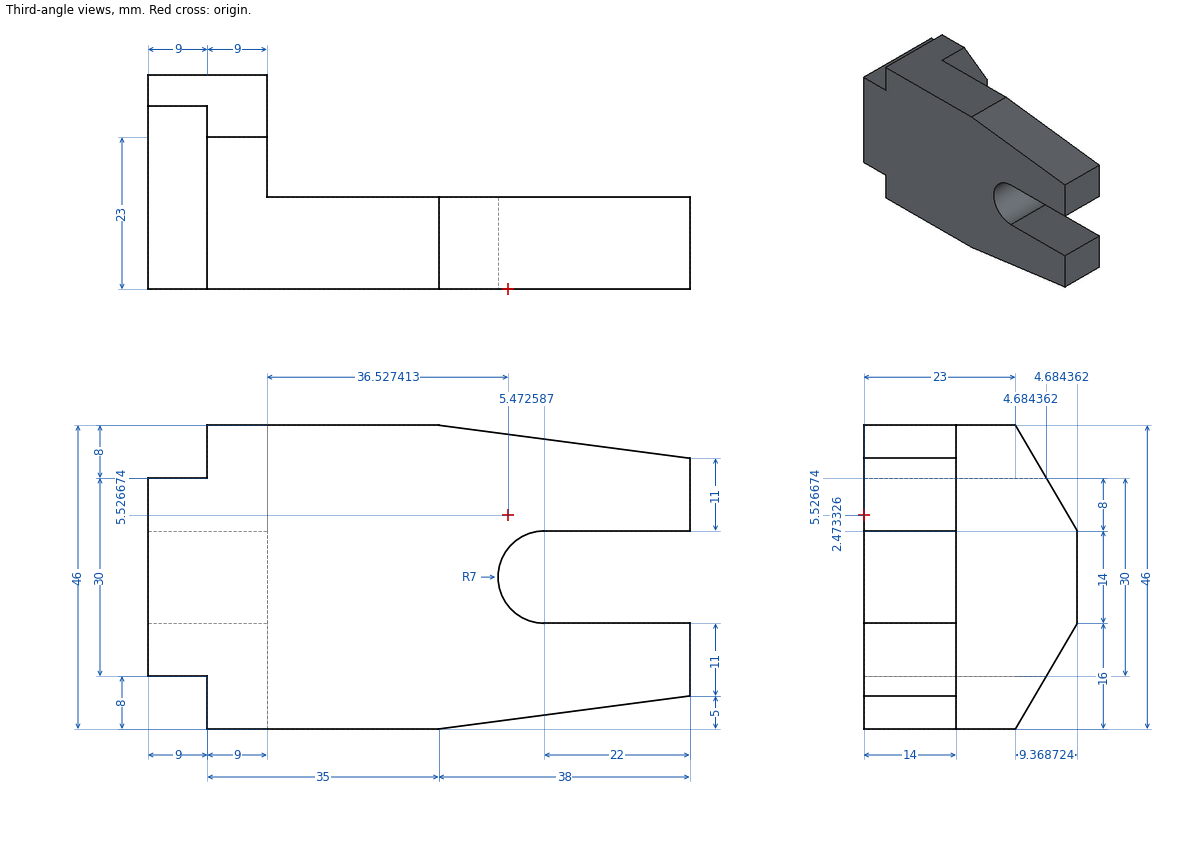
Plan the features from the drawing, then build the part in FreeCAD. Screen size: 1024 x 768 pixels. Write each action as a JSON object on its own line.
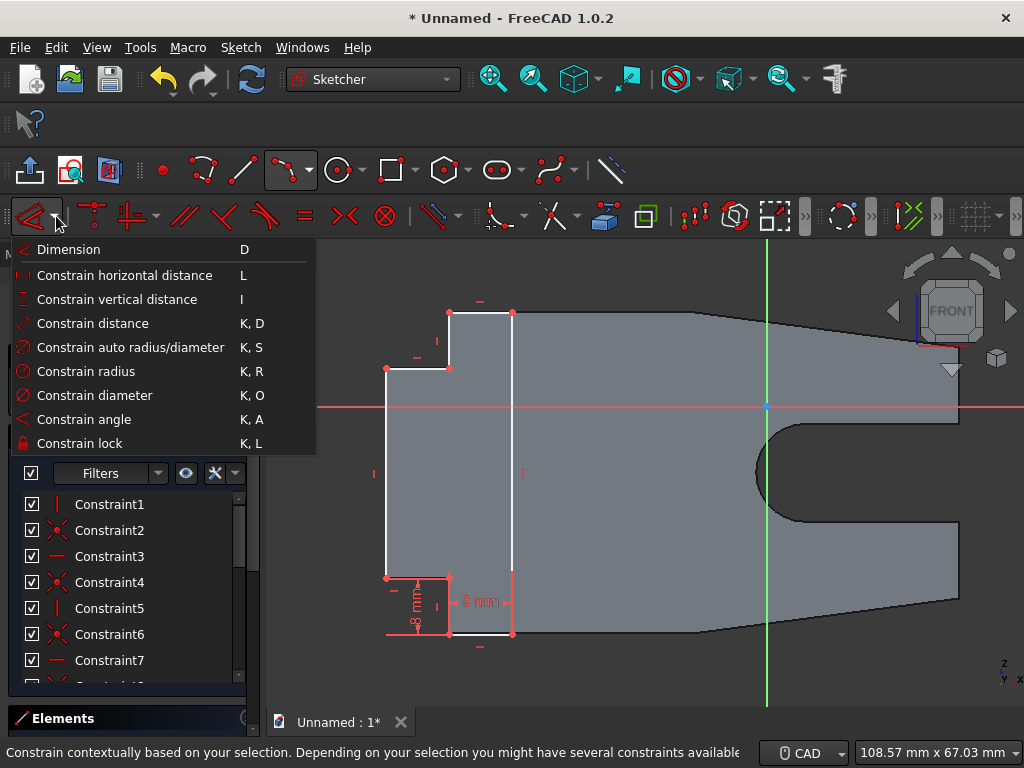
{"action": "left_click", "coordinate": [164, 275]}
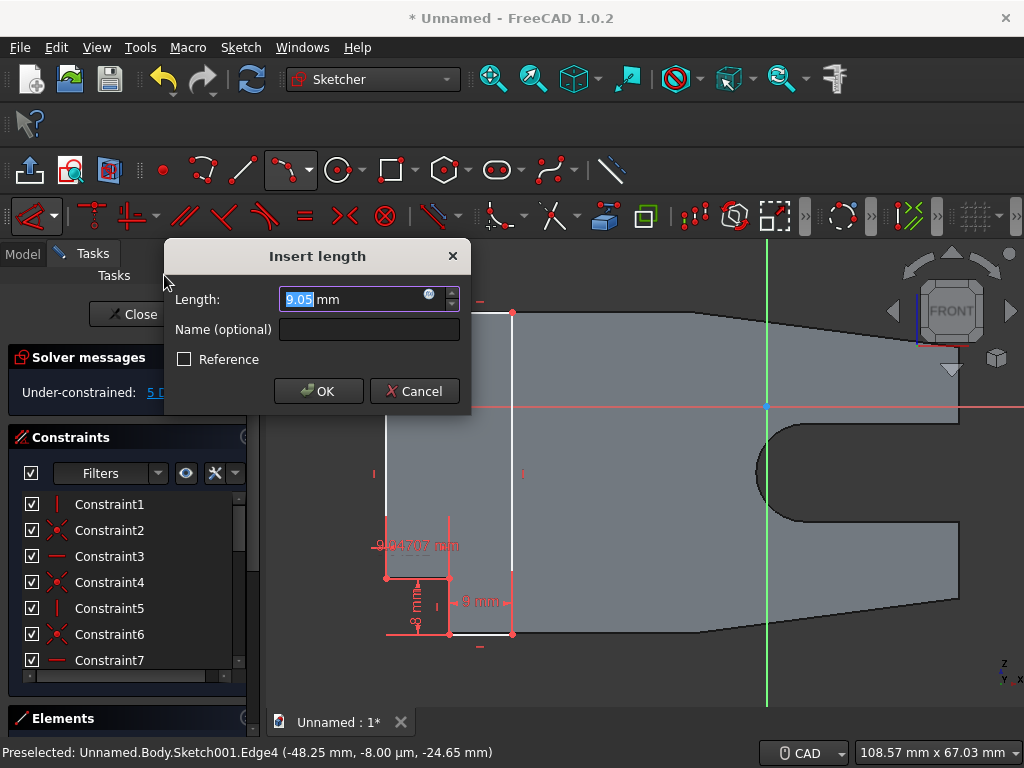
{"action": "type", "text": "9"}
{"action": "key", "text": "Return"}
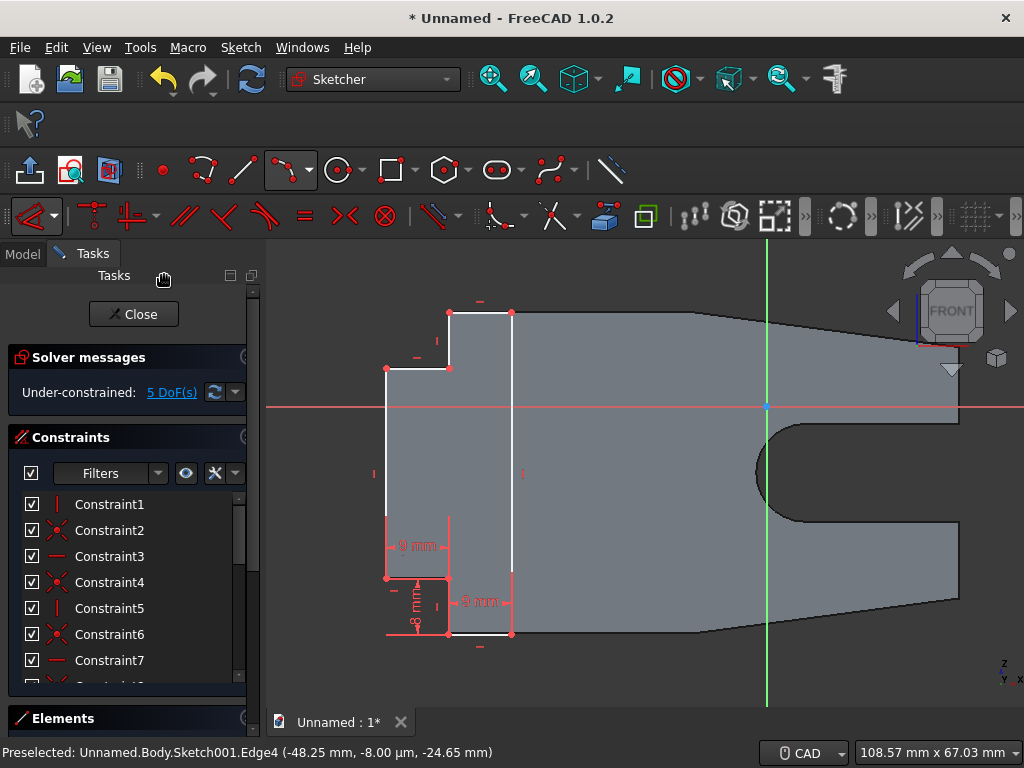
{"action": "left_click", "coordinate": [405, 369]}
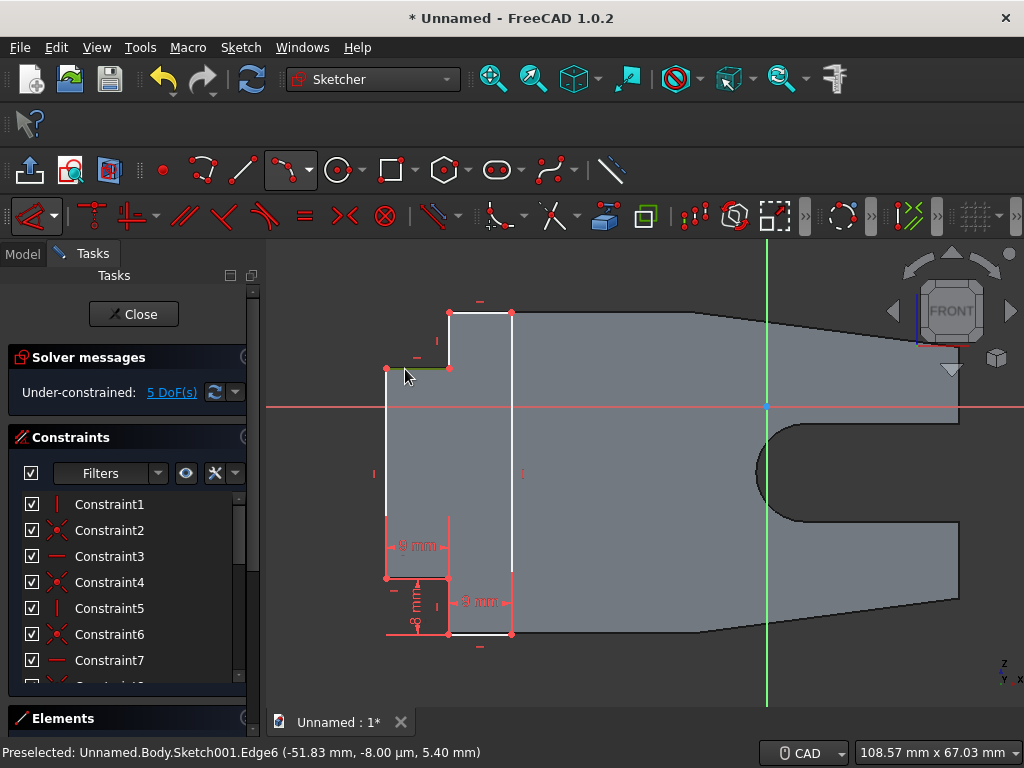
{"action": "left_click", "coordinate": [56, 216]}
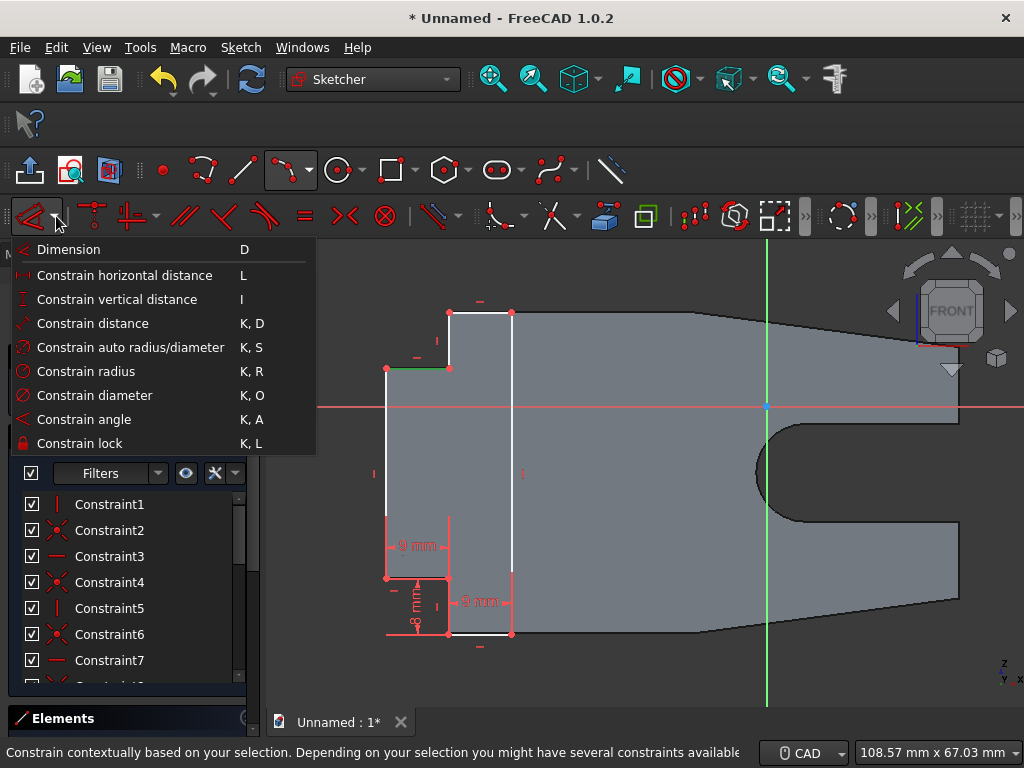
{"action": "left_click", "coordinate": [164, 275]}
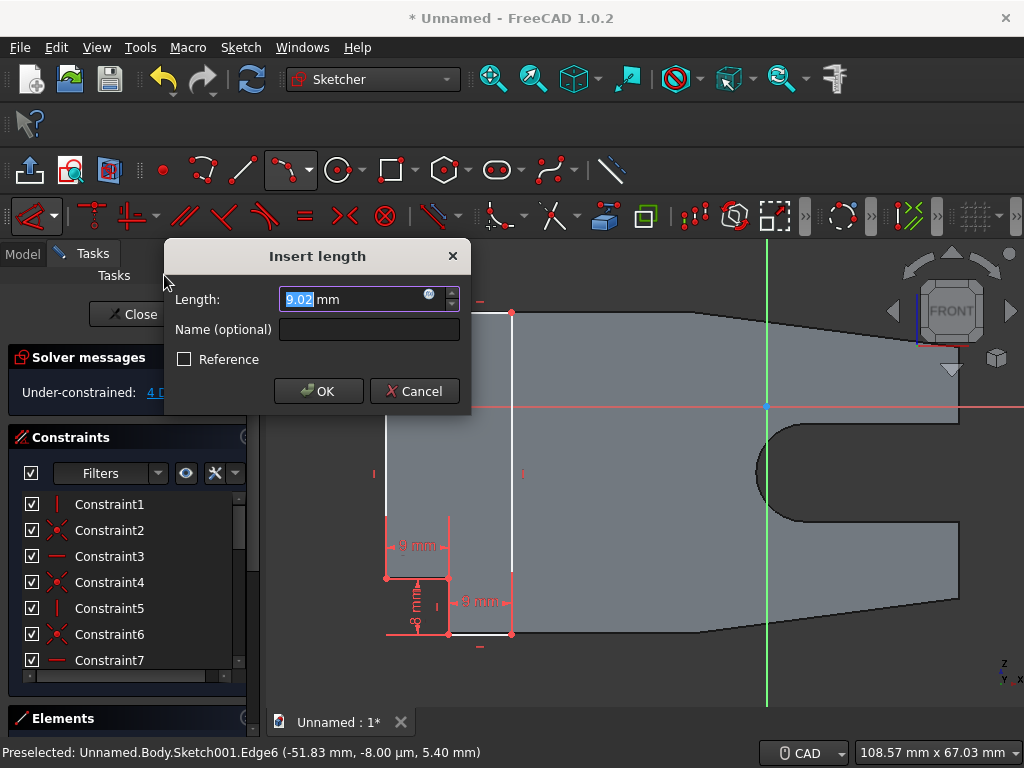
{"action": "type", "text": "9"}
{"action": "key", "text": "Return"}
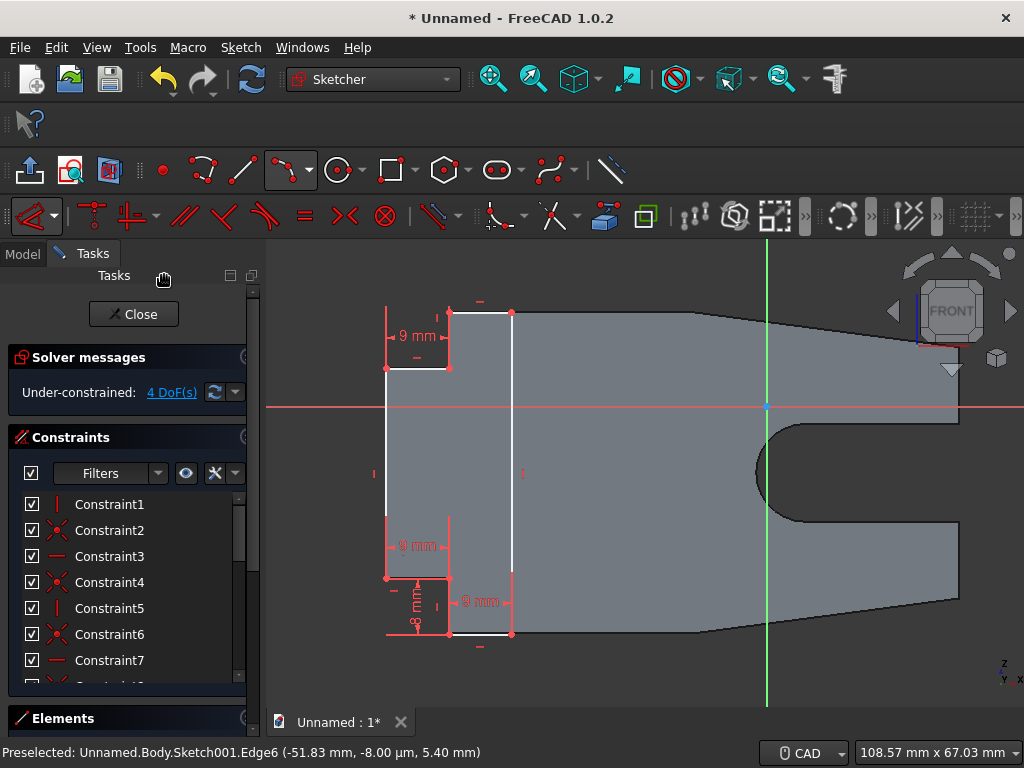
{"action": "left_click", "coordinate": [449, 352]}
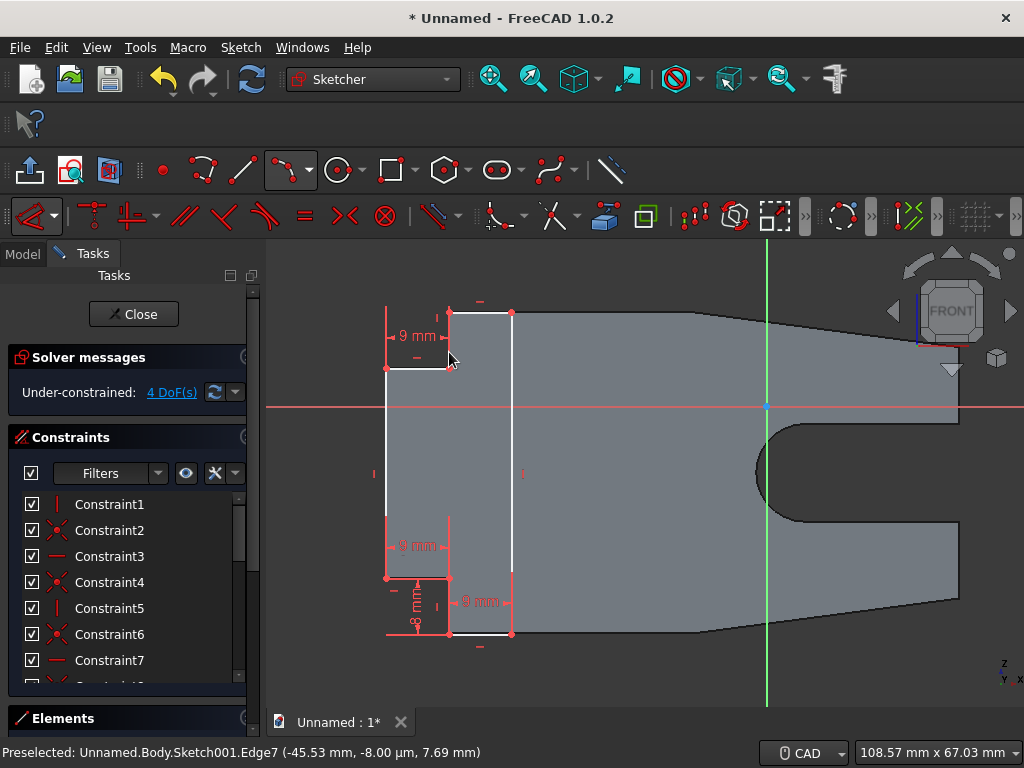
{"action": "left_click", "coordinate": [56, 216]}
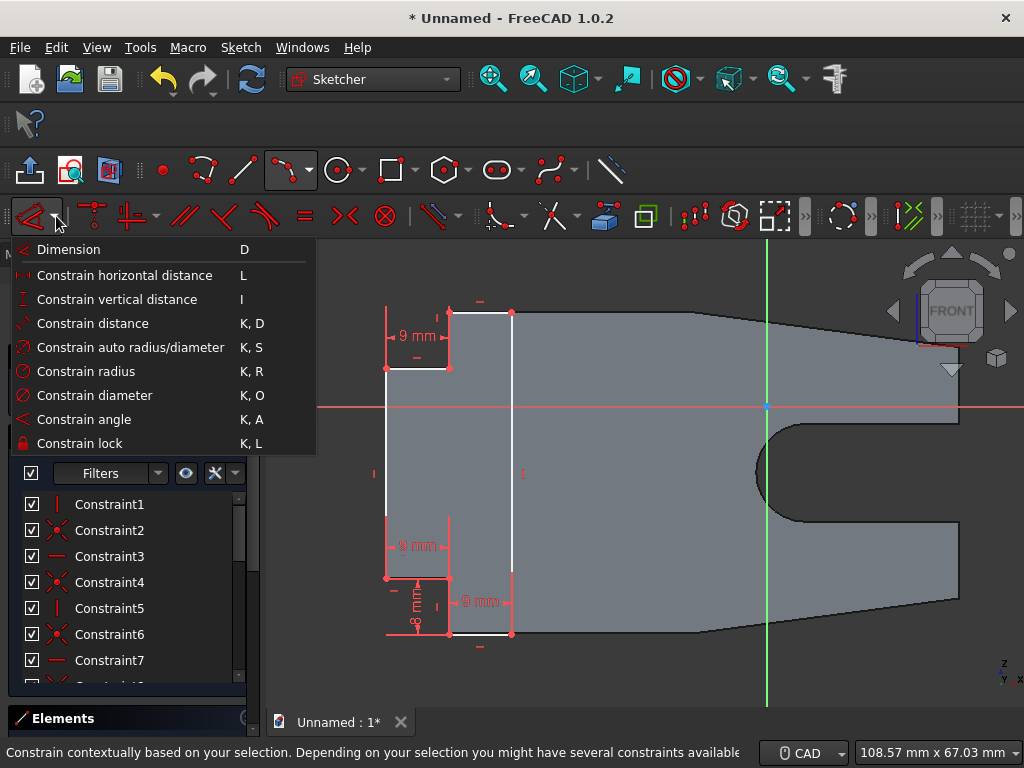
{"action": "left_click", "coordinate": [164, 299]}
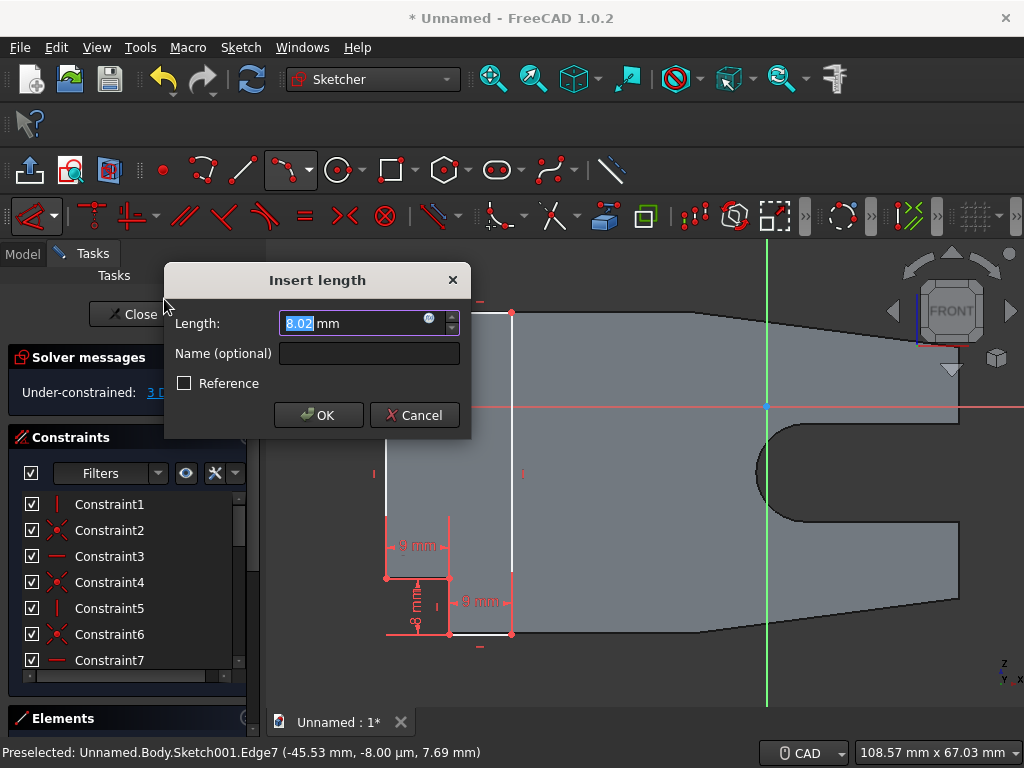
{"action": "type", "text": "8"}
{"action": "key", "text": "Return"}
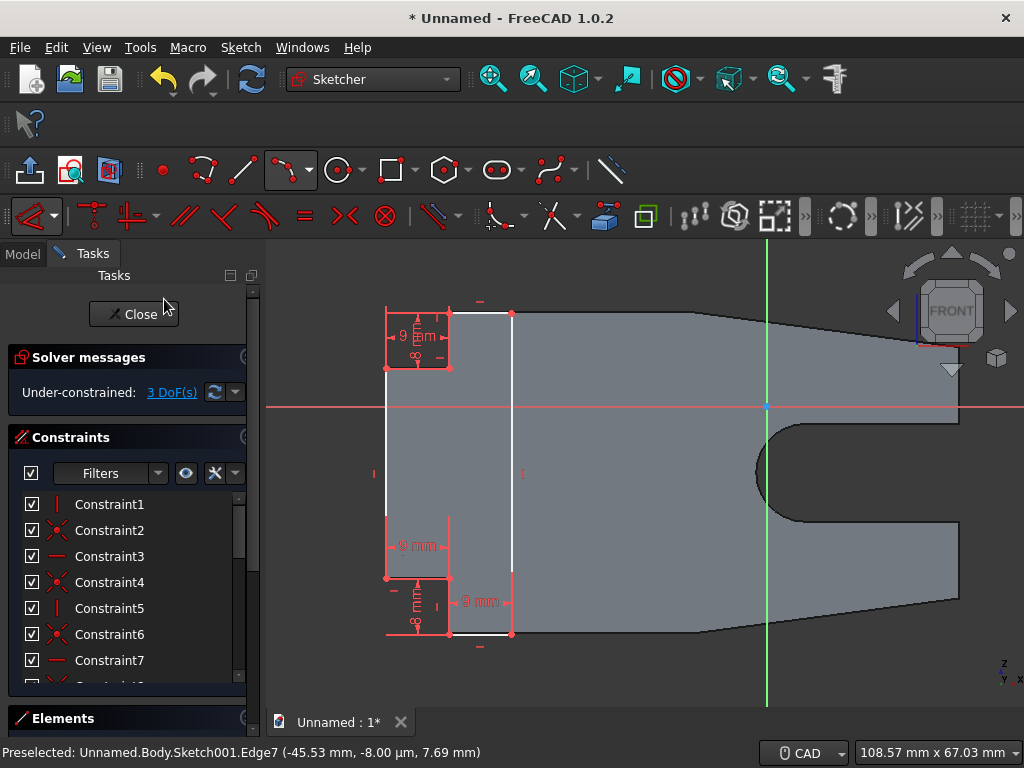
{"action": "left_click", "coordinate": [512, 410]}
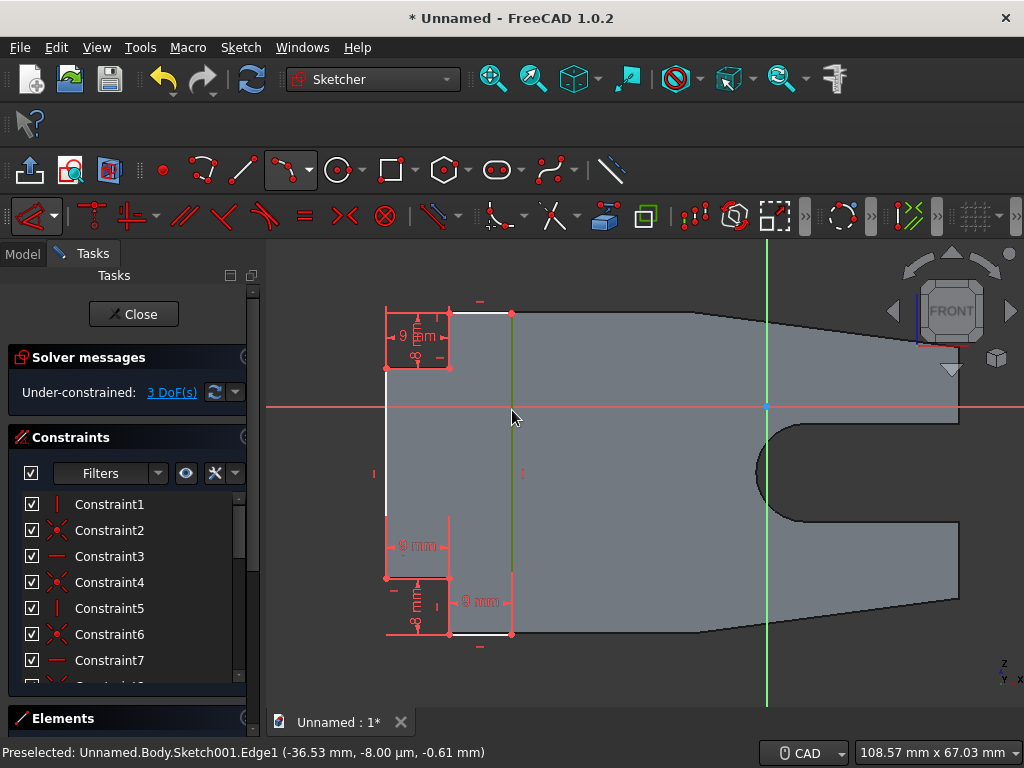
{"action": "left_click", "coordinate": [56, 216]}